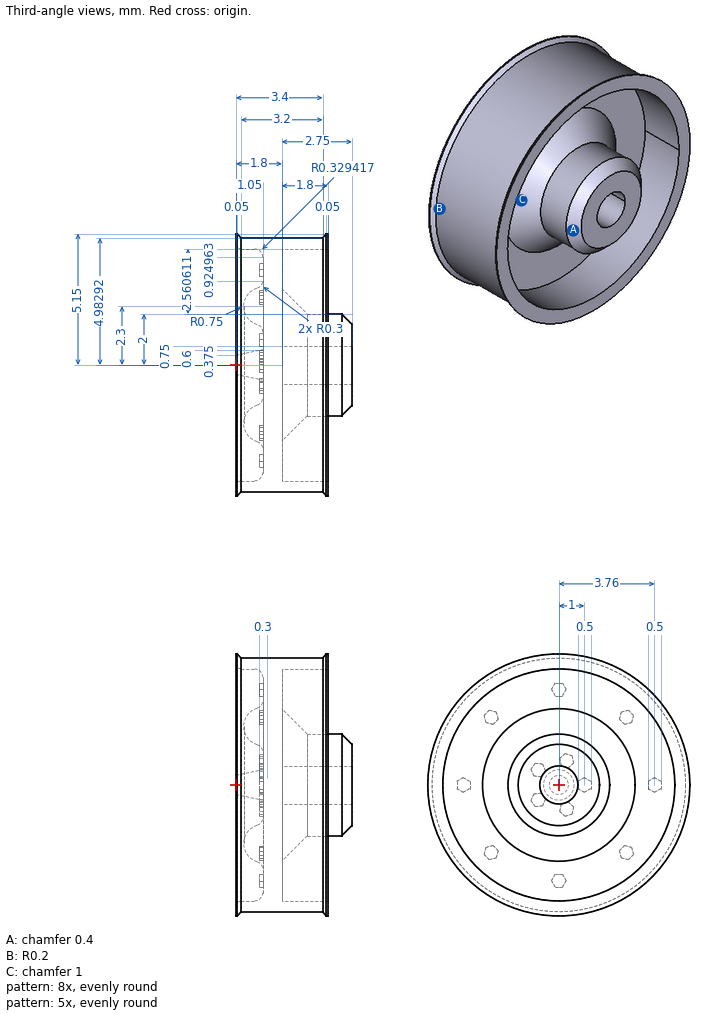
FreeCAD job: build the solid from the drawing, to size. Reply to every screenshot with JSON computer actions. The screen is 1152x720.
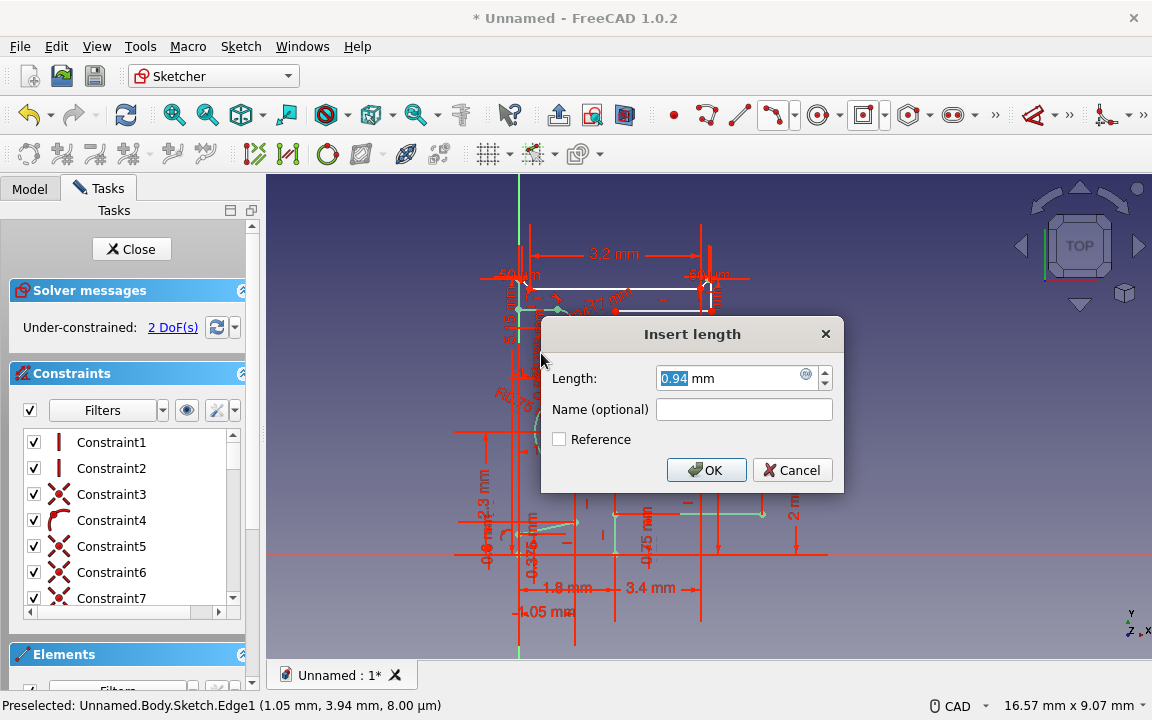
{"action": "type", "text": "0.924963"}
{"action": "key", "text": "Return"}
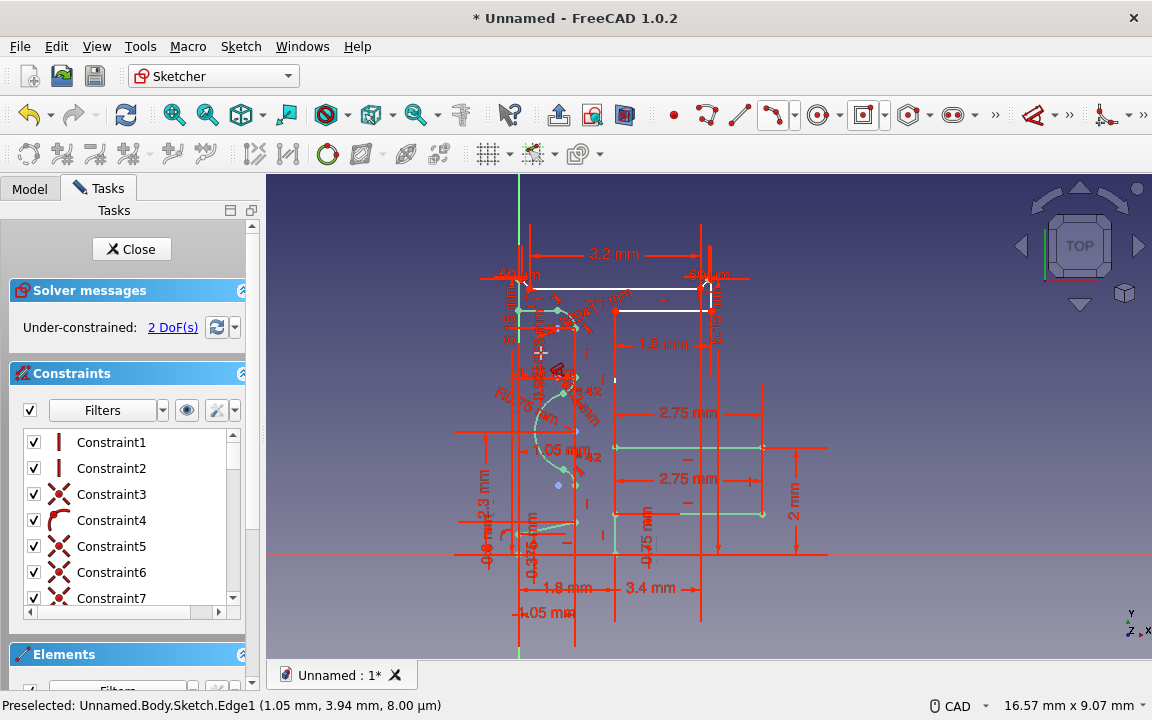
{"action": "left_click", "coordinate": [615, 407]}
{"action": "left_click", "coordinate": [581, 427]}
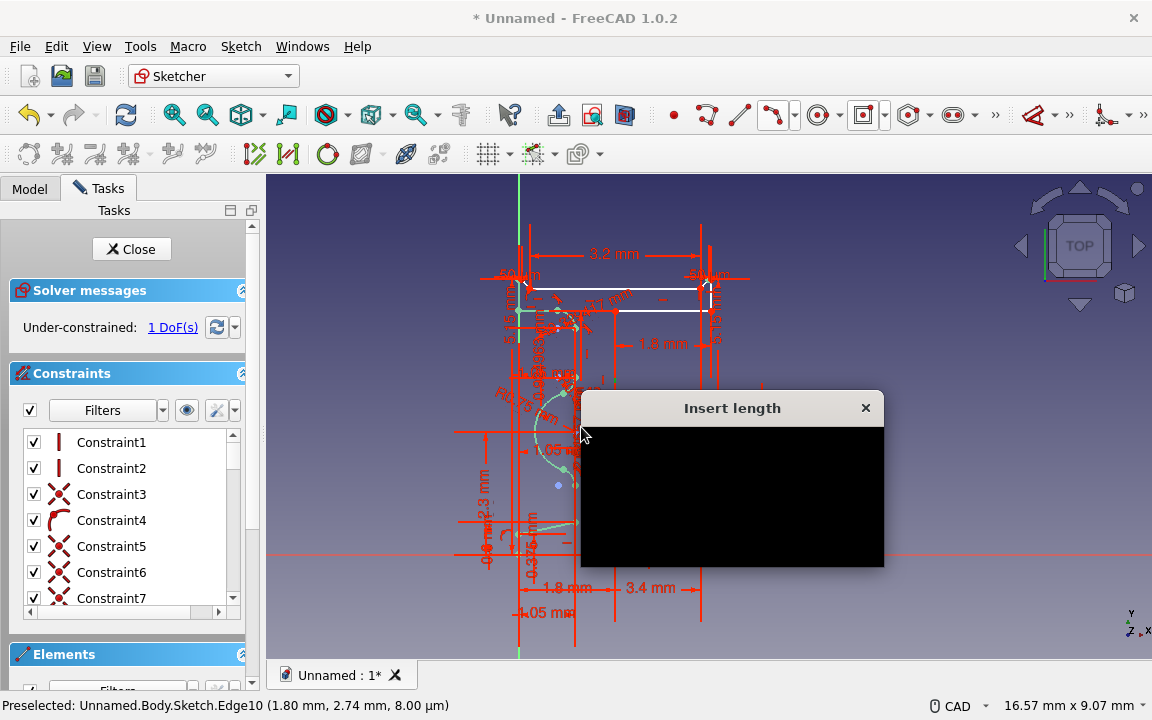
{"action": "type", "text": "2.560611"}
{"action": "key", "text": "Return"}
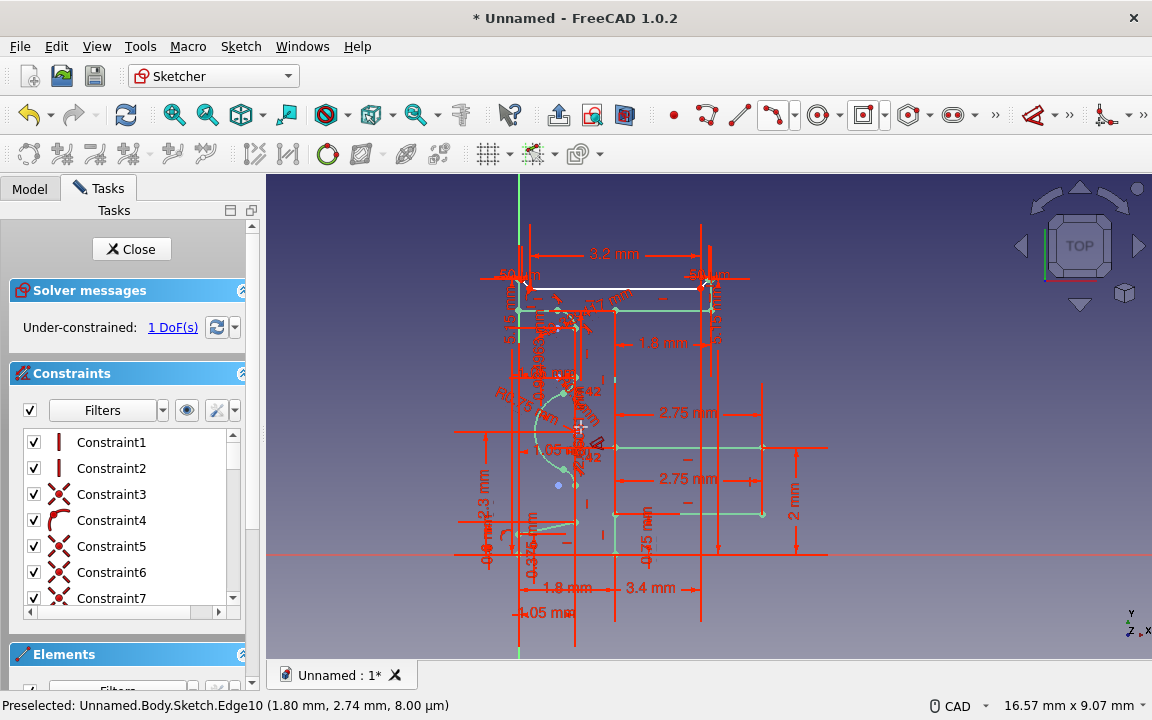
{"action": "left_click", "coordinate": [701, 289]}
{"action": "left_click", "coordinate": [485, 515]}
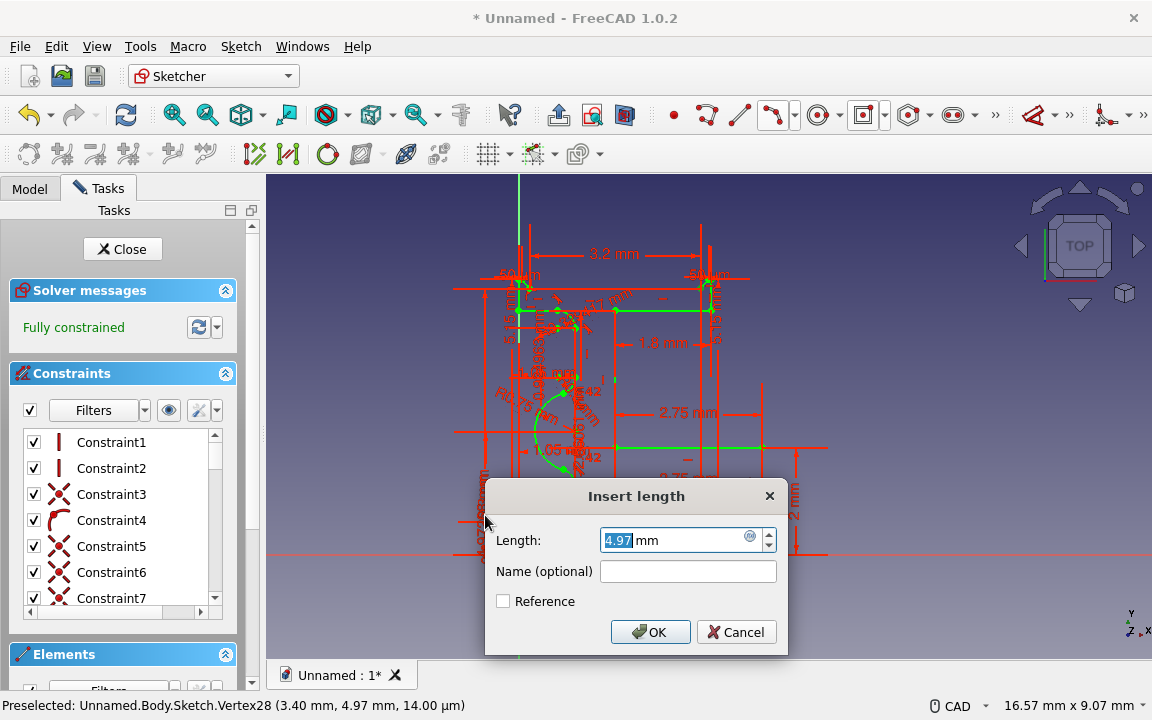
{"action": "type", "text": "4.98292"}
{"action": "key", "text": "Return"}
{"action": "key", "text": "Escape"}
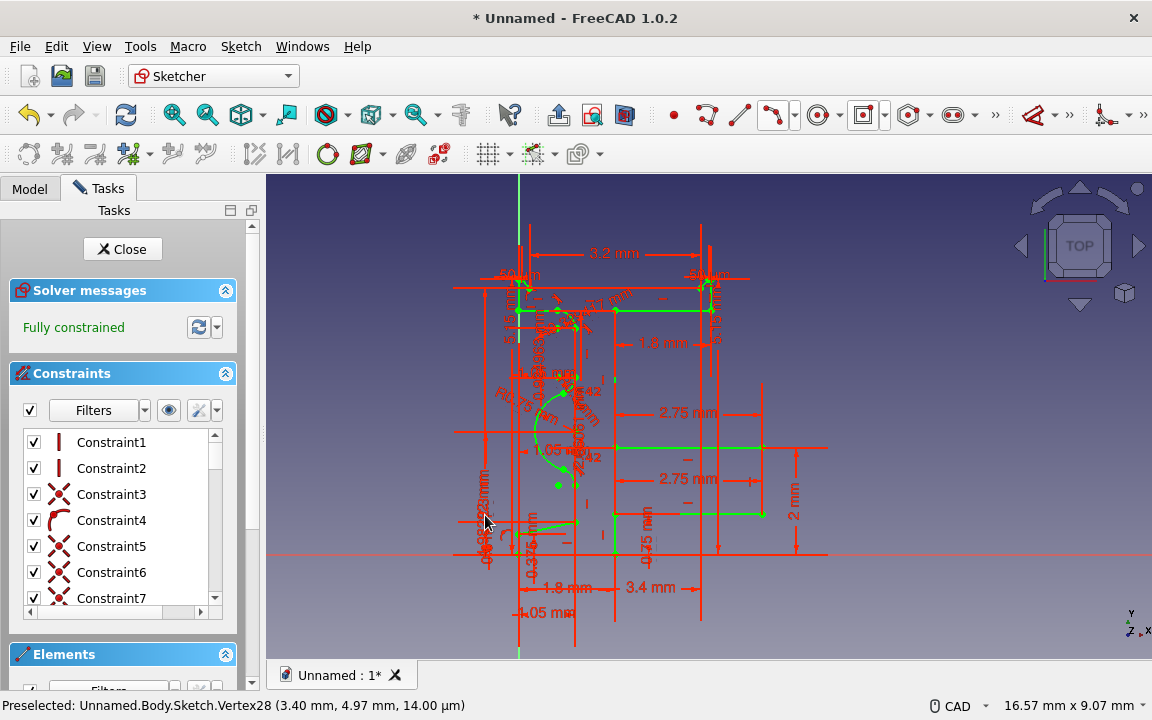
{"action": "left_click", "coordinate": [123, 249]}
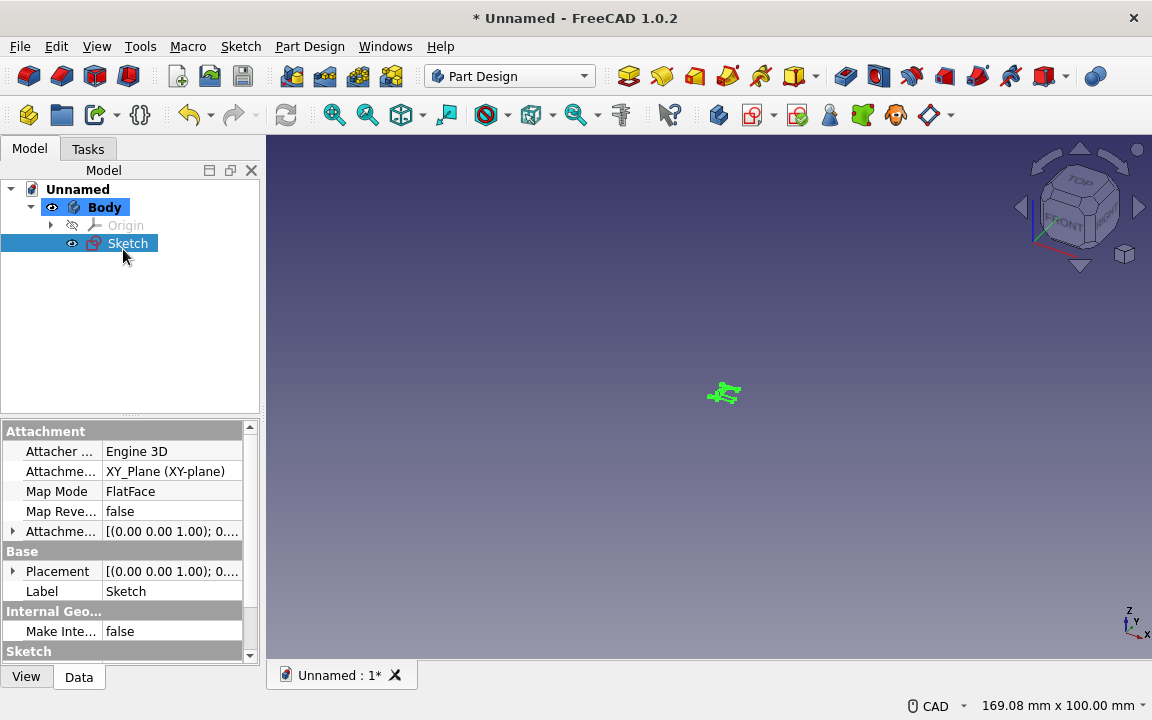
{"action": "left_click", "coordinate": [662, 76]}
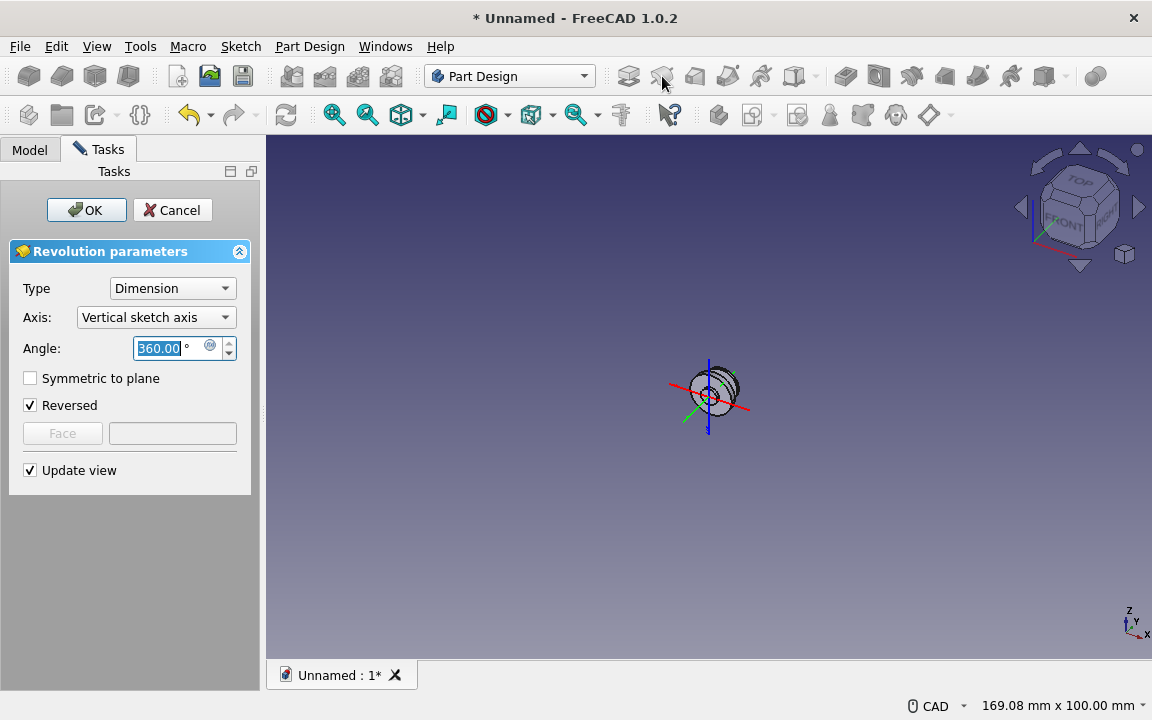
{"action": "left_click", "coordinate": [157, 318]}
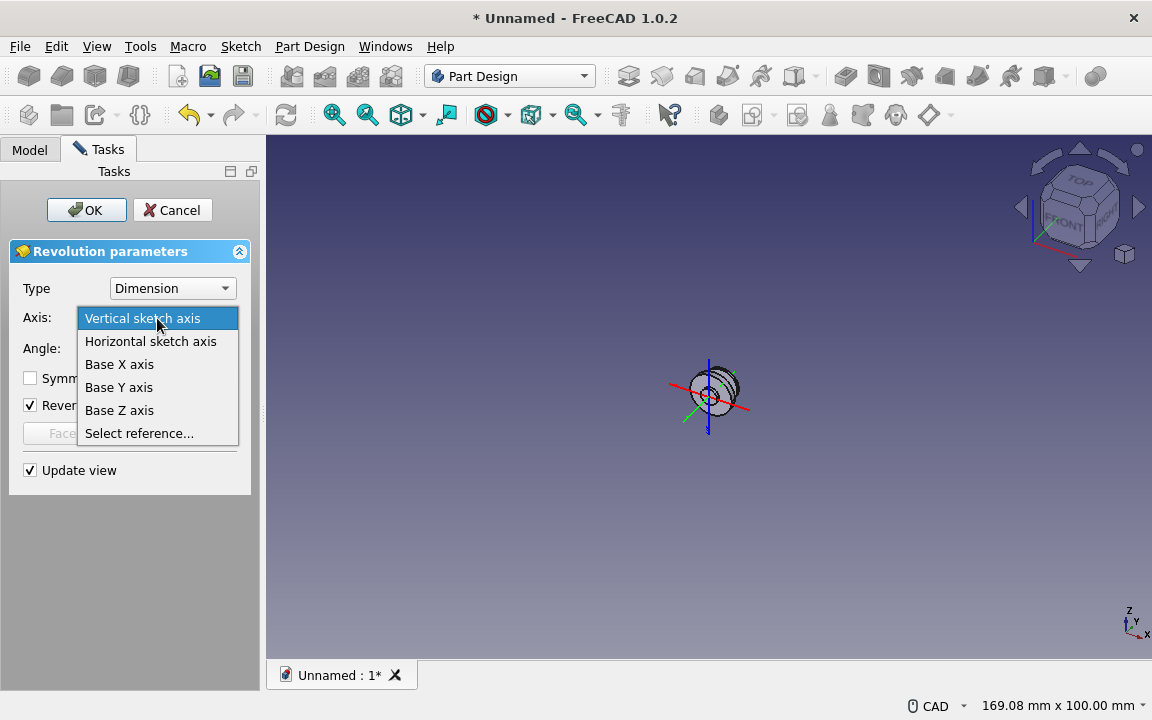
{"action": "left_click", "coordinate": [156, 342]}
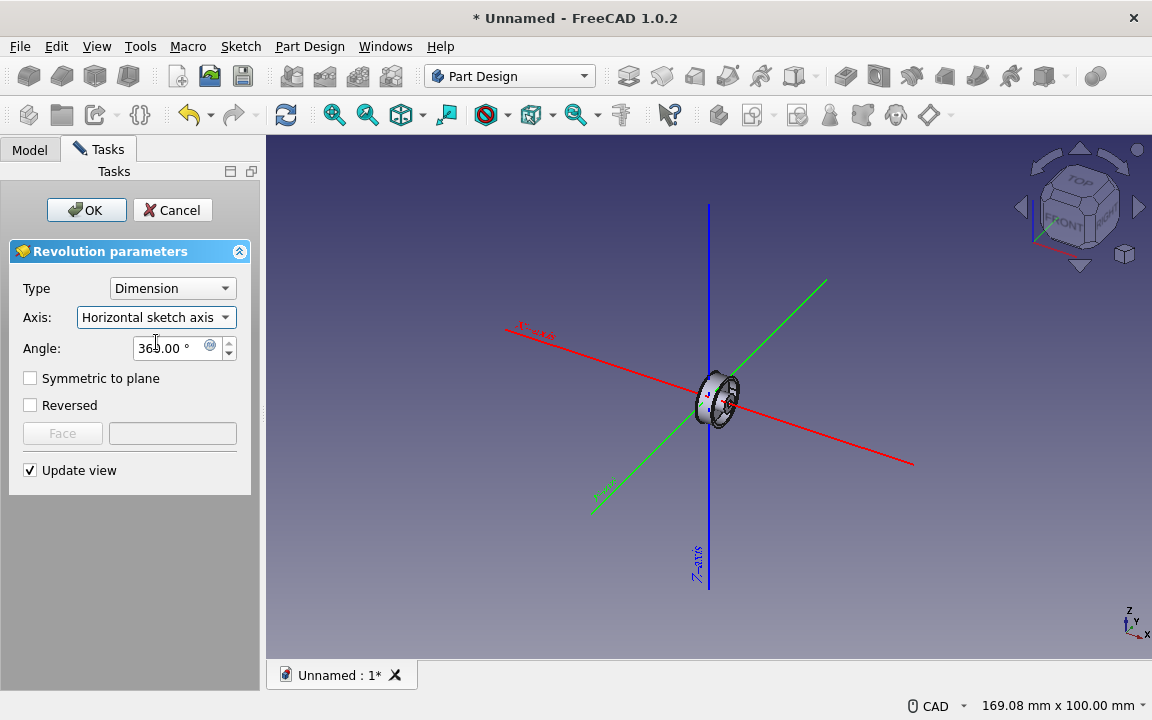
{"action": "left_click", "coordinate": [87, 210]}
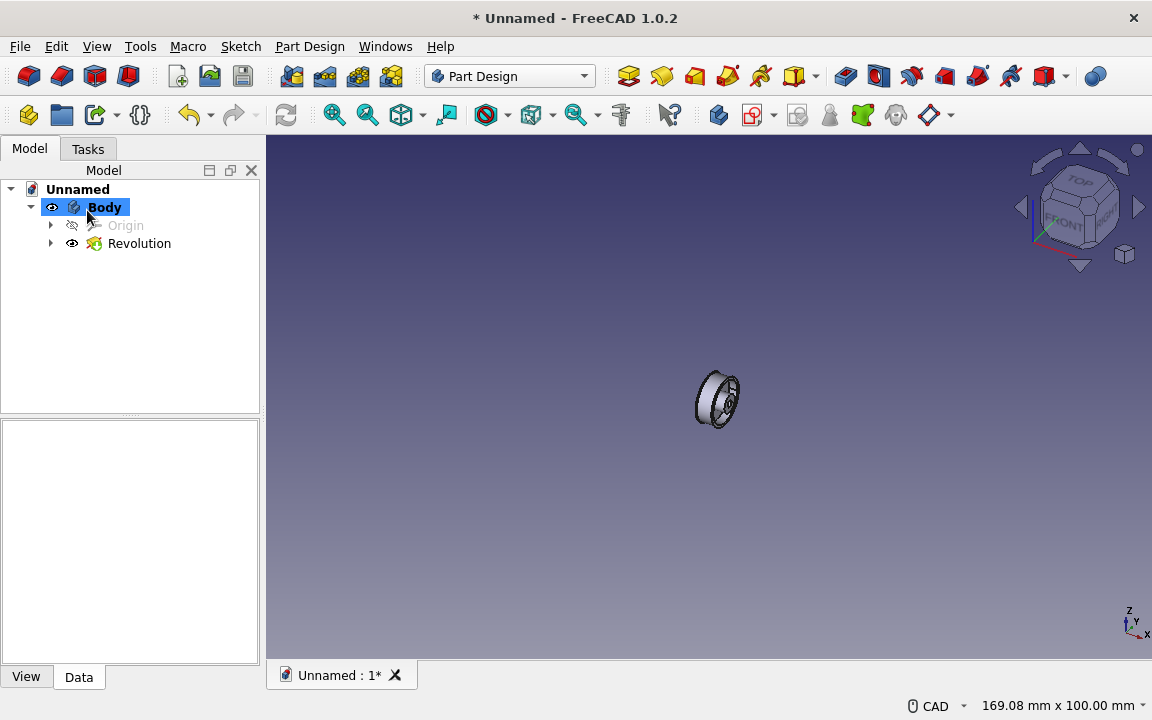
{"action": "left_click", "coordinate": [335, 116]}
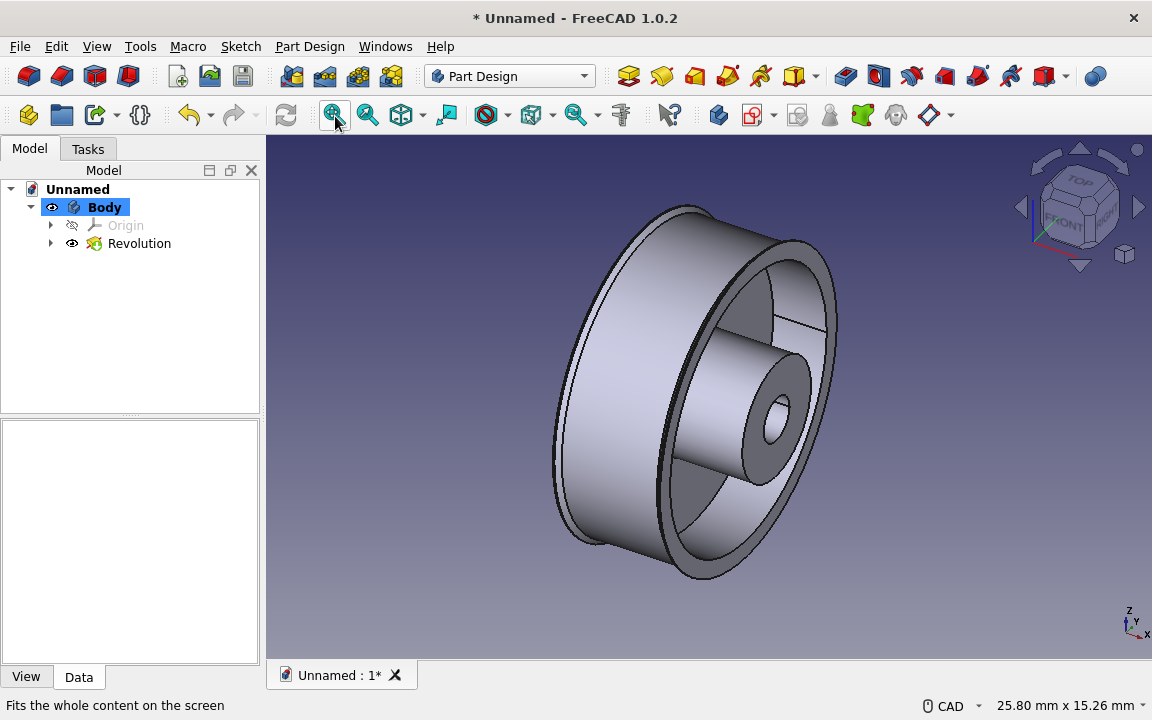
{"action": "left_click", "coordinate": [742, 453]}